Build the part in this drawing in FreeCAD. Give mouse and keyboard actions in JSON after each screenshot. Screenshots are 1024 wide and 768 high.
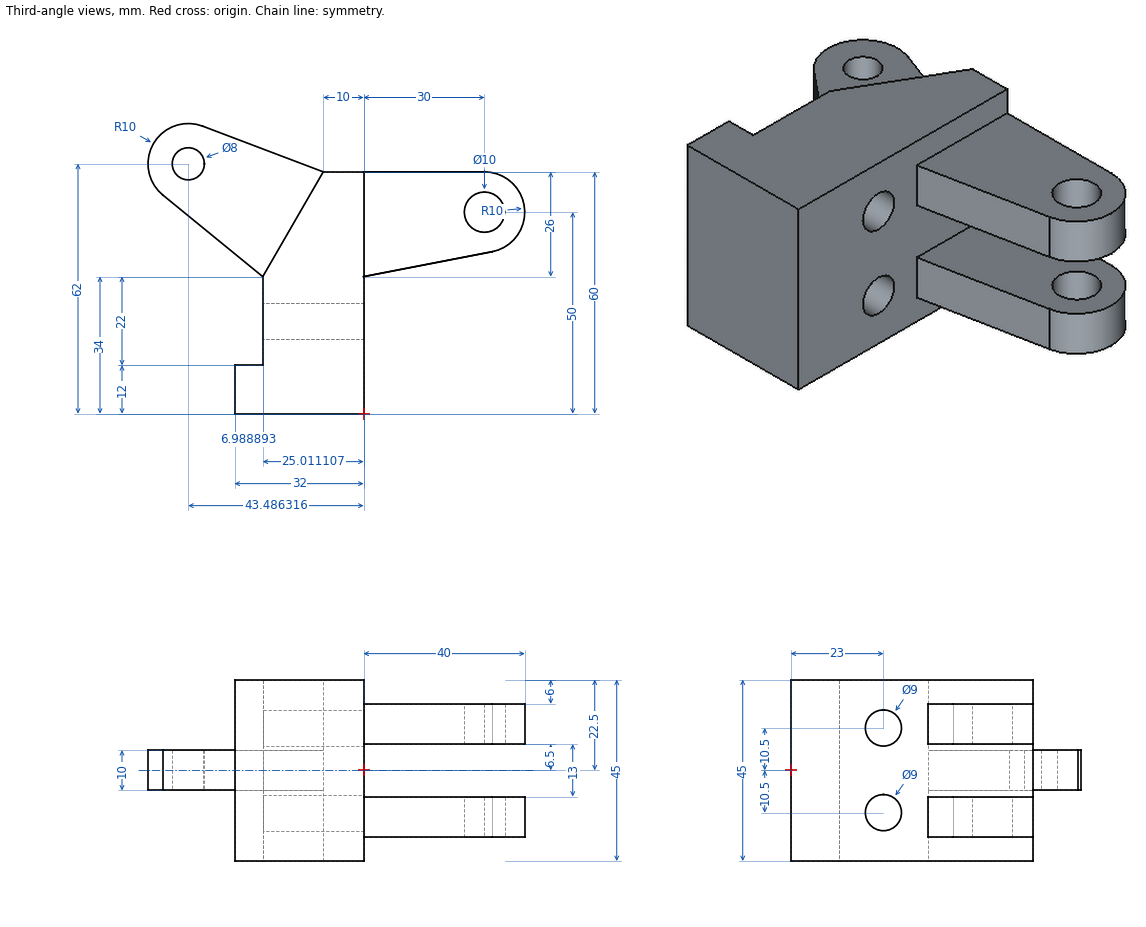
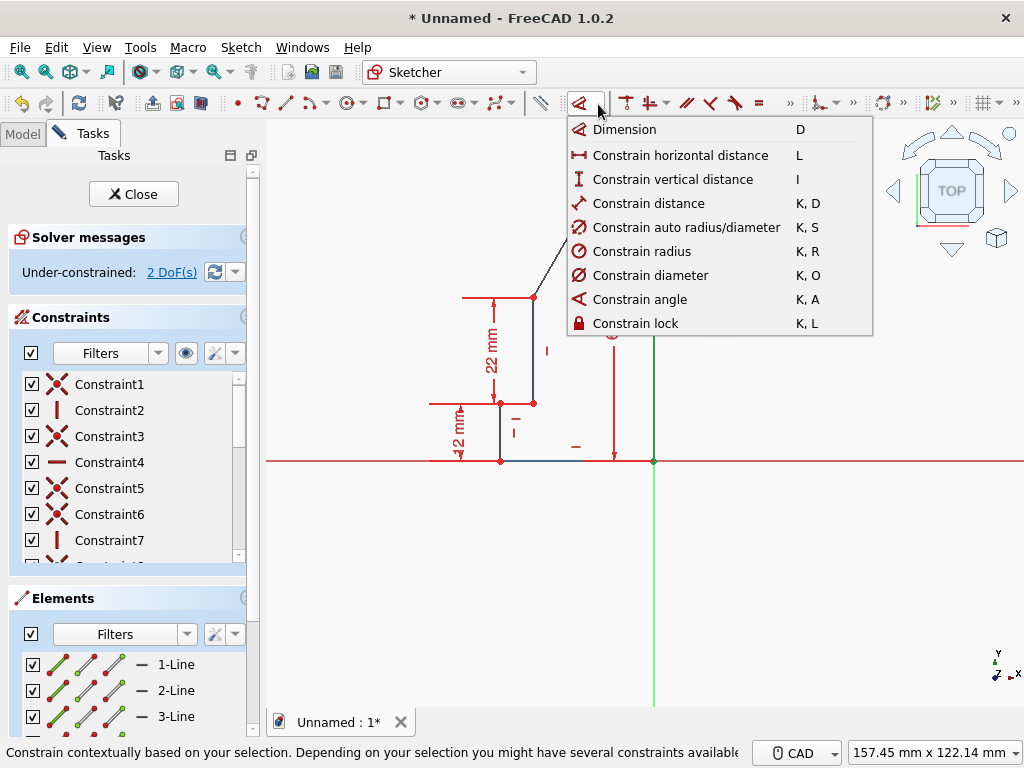
{"action": "left_click", "coordinate": [720, 155]}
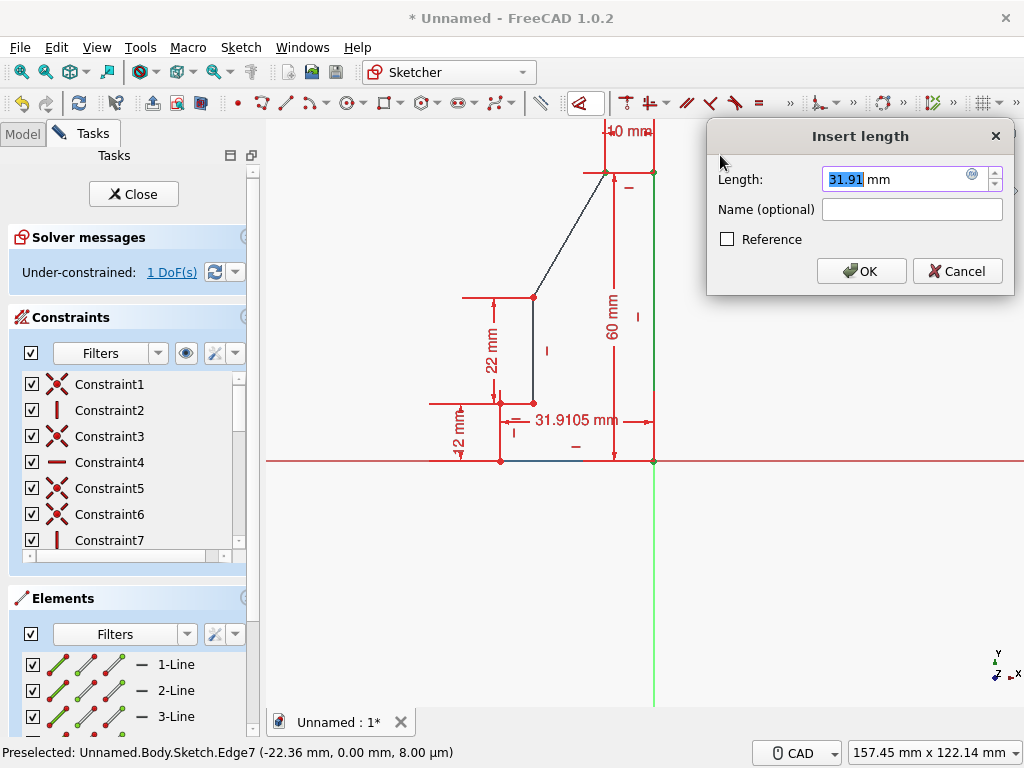
{"action": "type", "text": "32"}
{"action": "key", "text": "Return"}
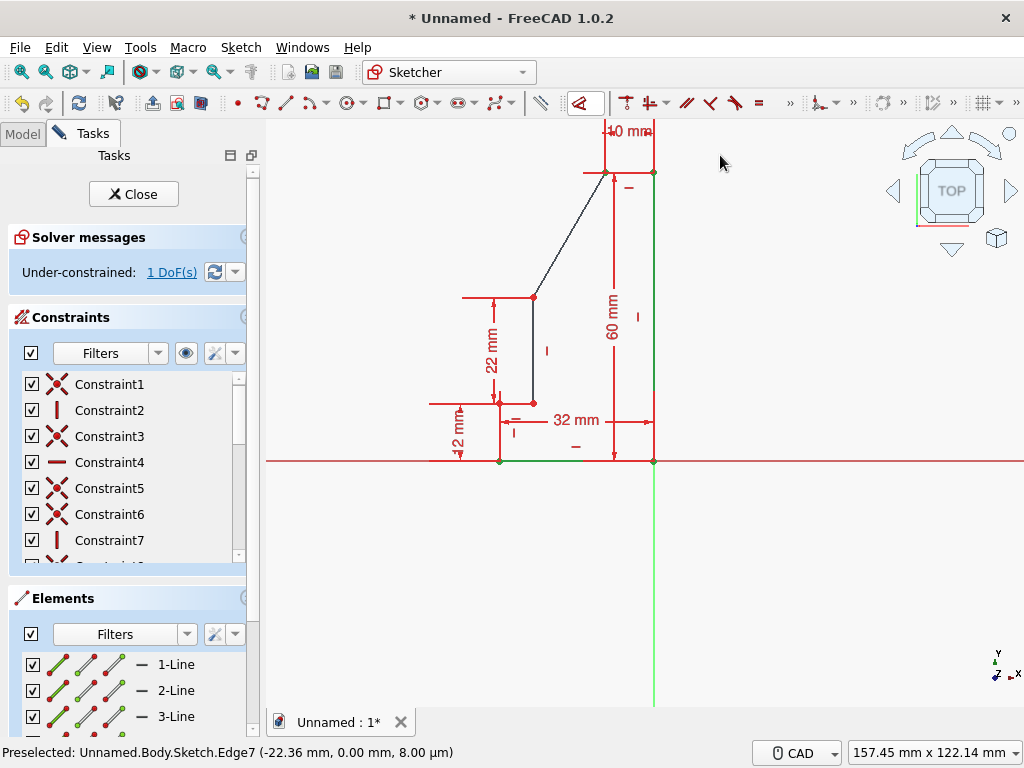
{"action": "scroll", "coordinate": [523, 404], "scroll_direction": "up", "scroll_amount": 2}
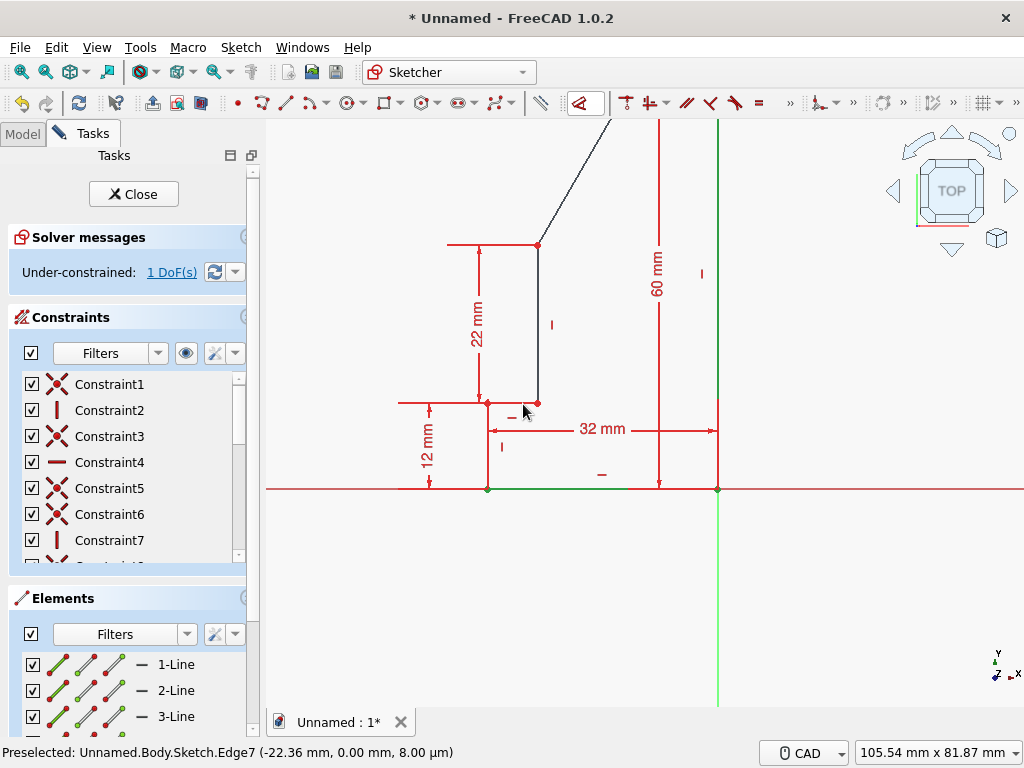
{"action": "left_click", "coordinate": [523, 403]}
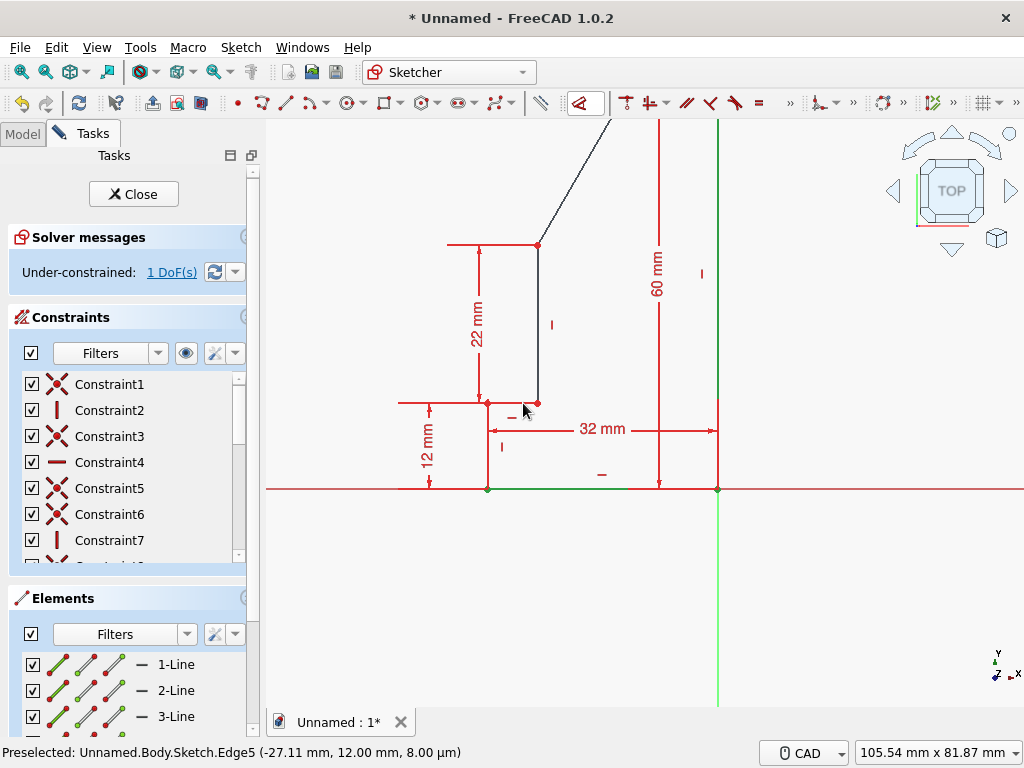
{"action": "key", "text": "l"}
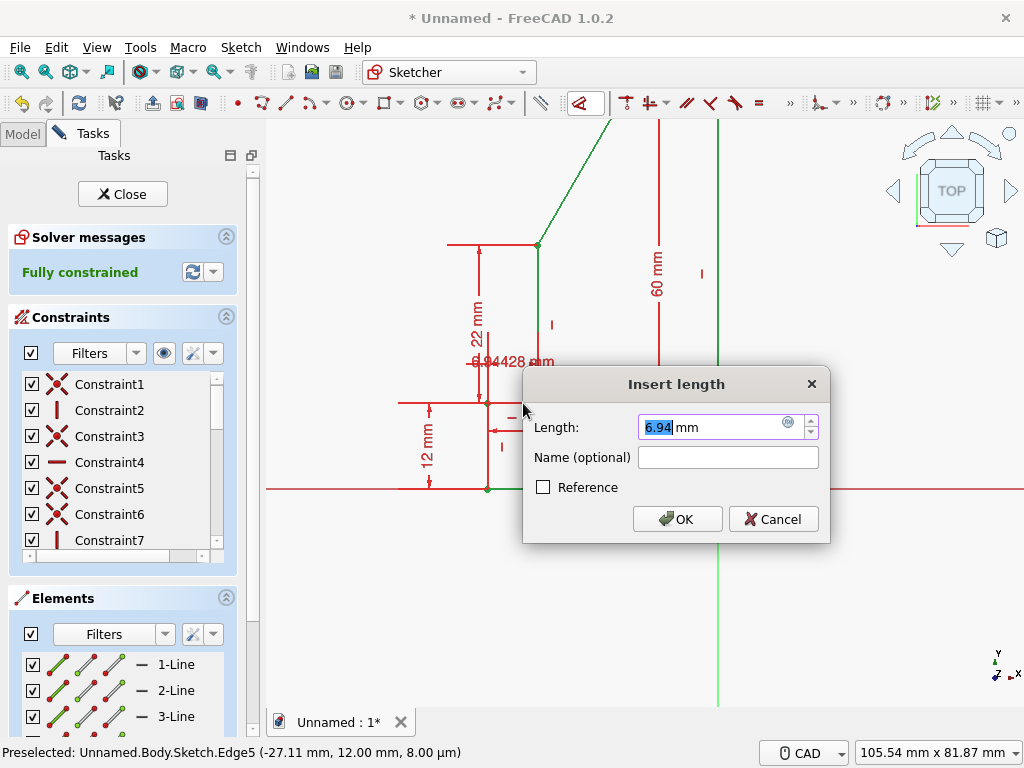
{"action": "type", "text": "6.988893"}
{"action": "key", "text": "Return"}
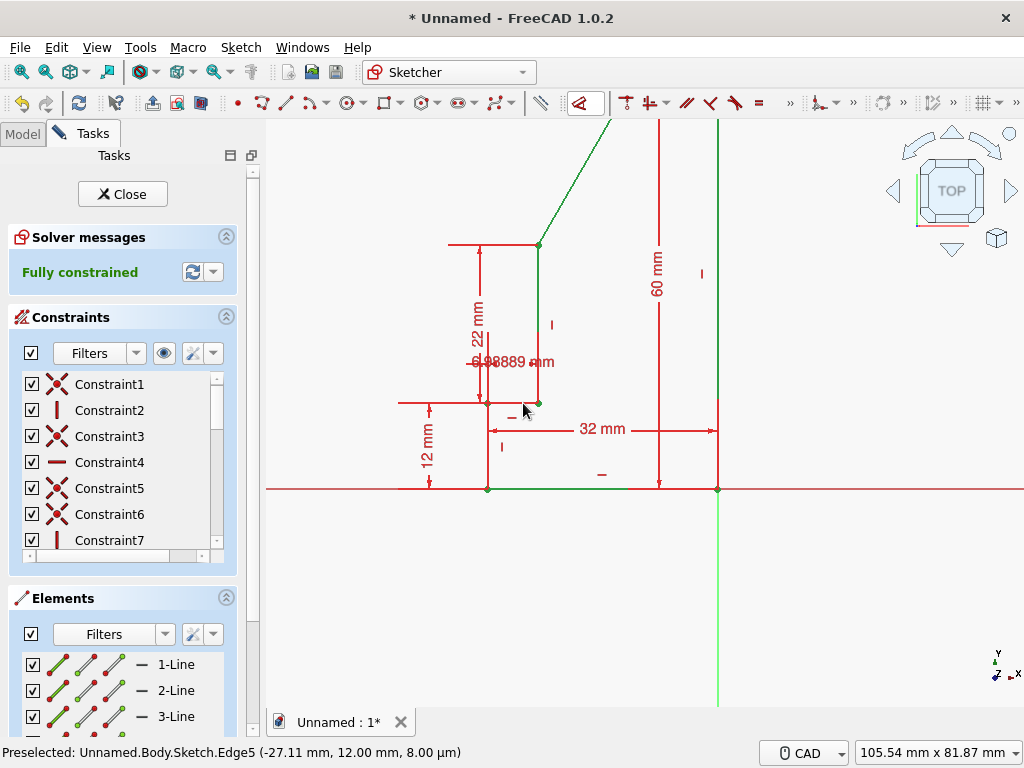
{"action": "left_click", "coordinate": [123, 194]}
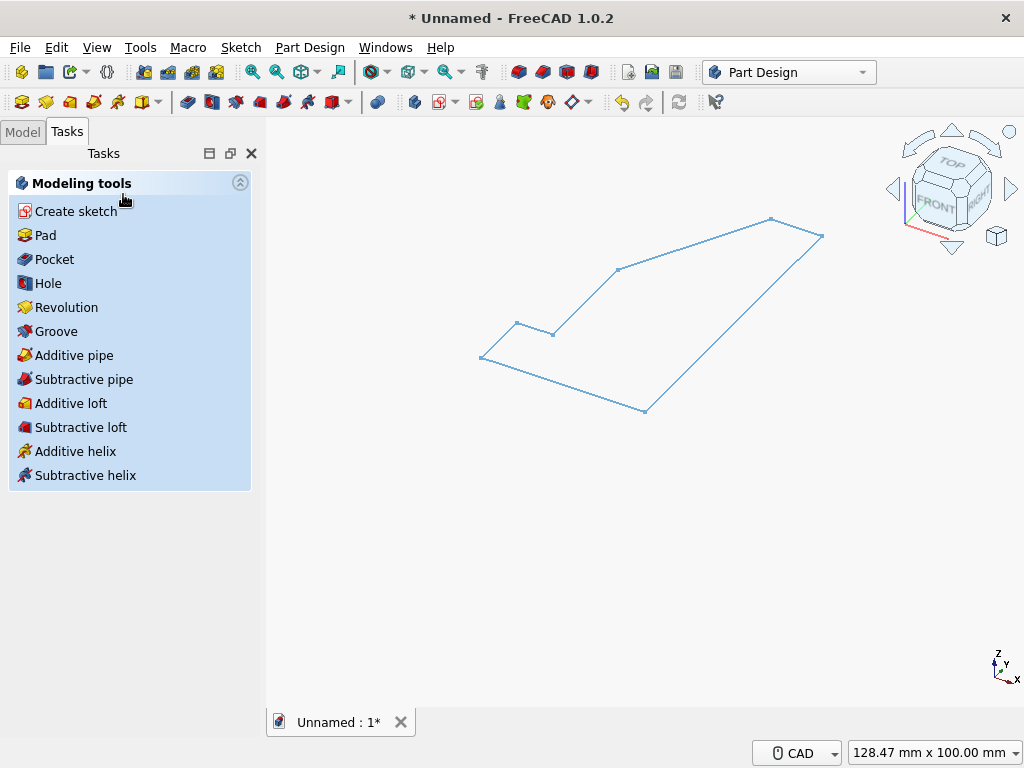
{"action": "left_click", "coordinate": [22, 102]}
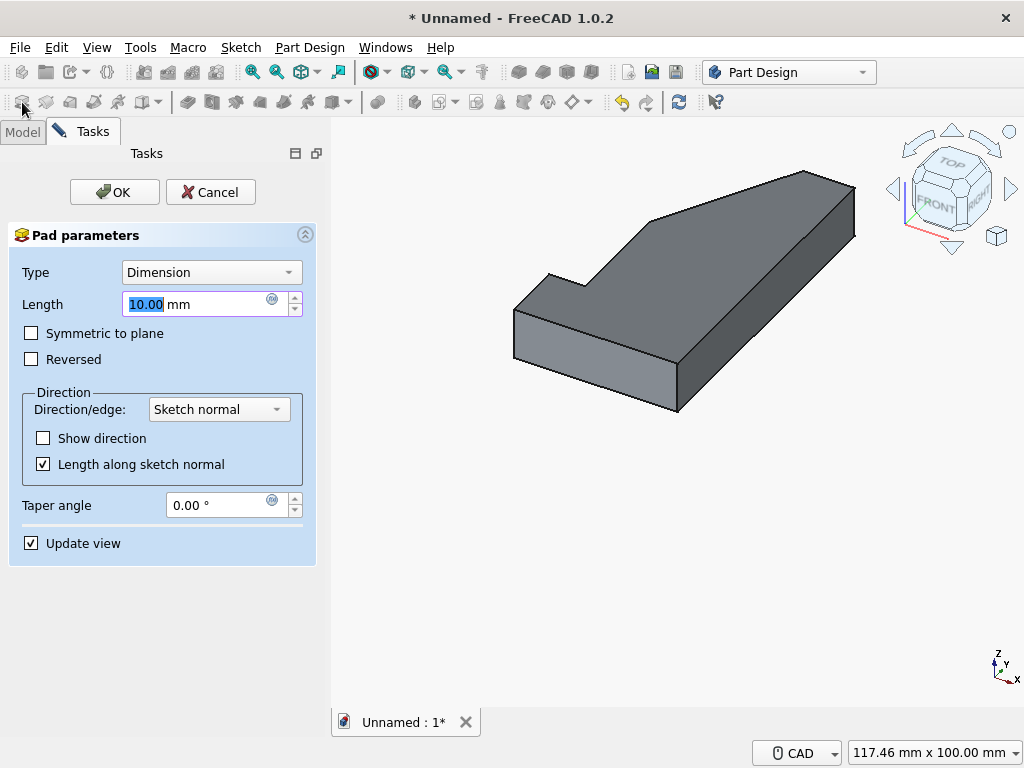
{"action": "type", "text": "45"}
{"action": "key", "text": "Tab"}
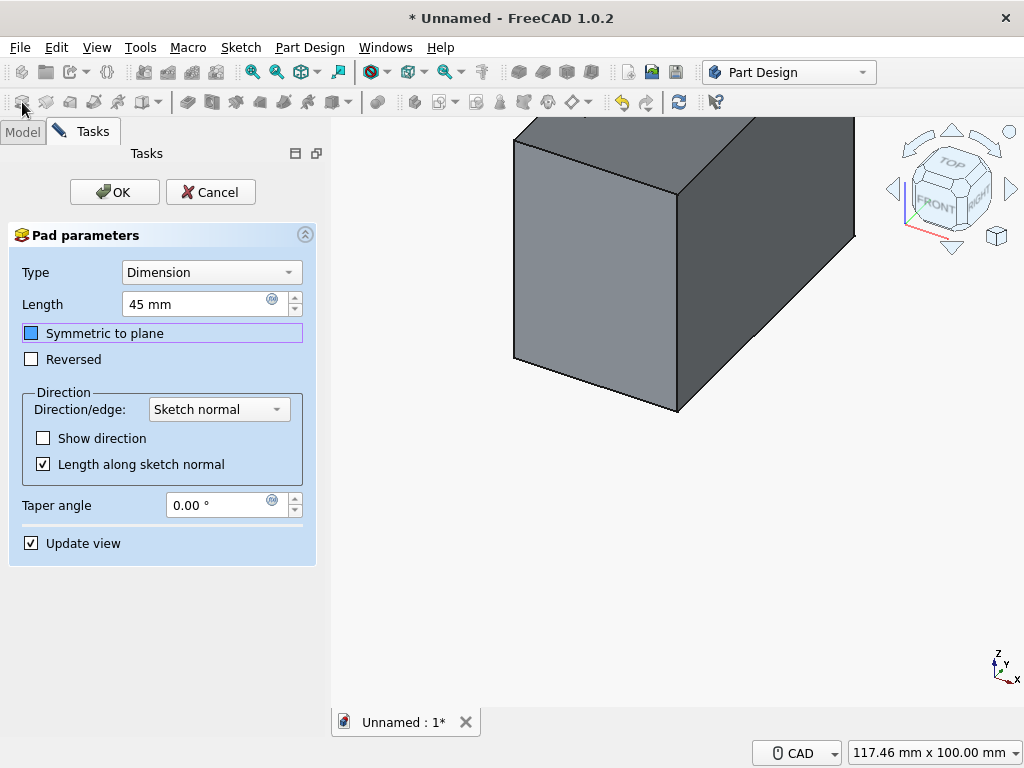
{"action": "left_click", "coordinate": [30, 333]}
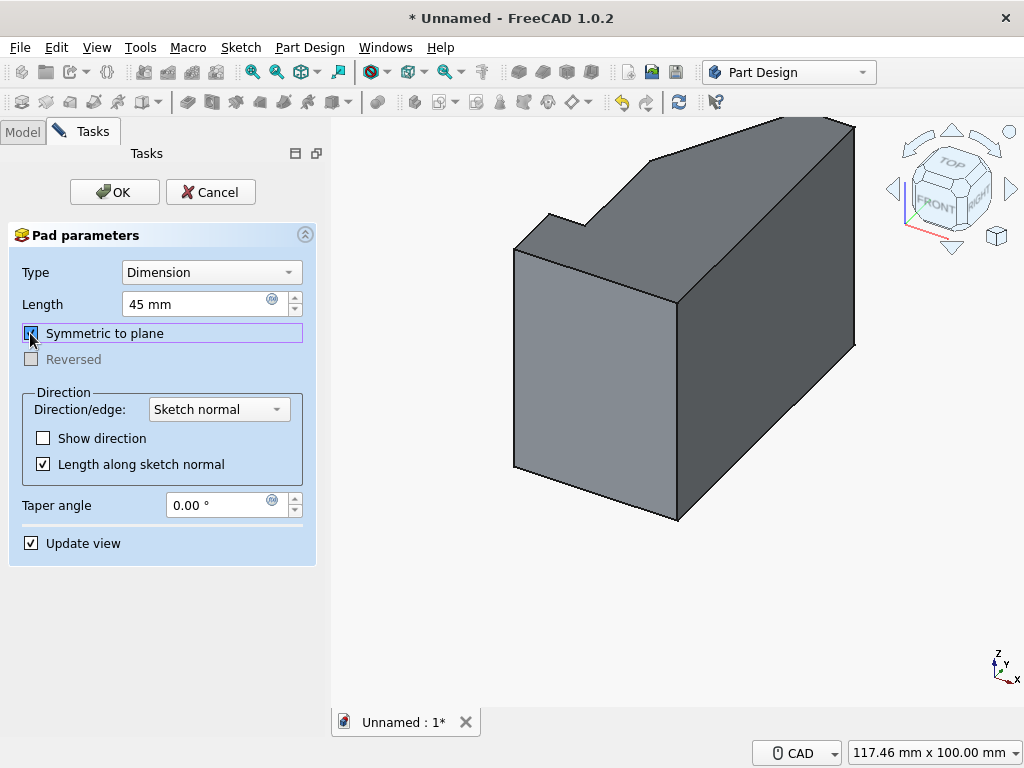
{"action": "left_click", "coordinate": [115, 192]}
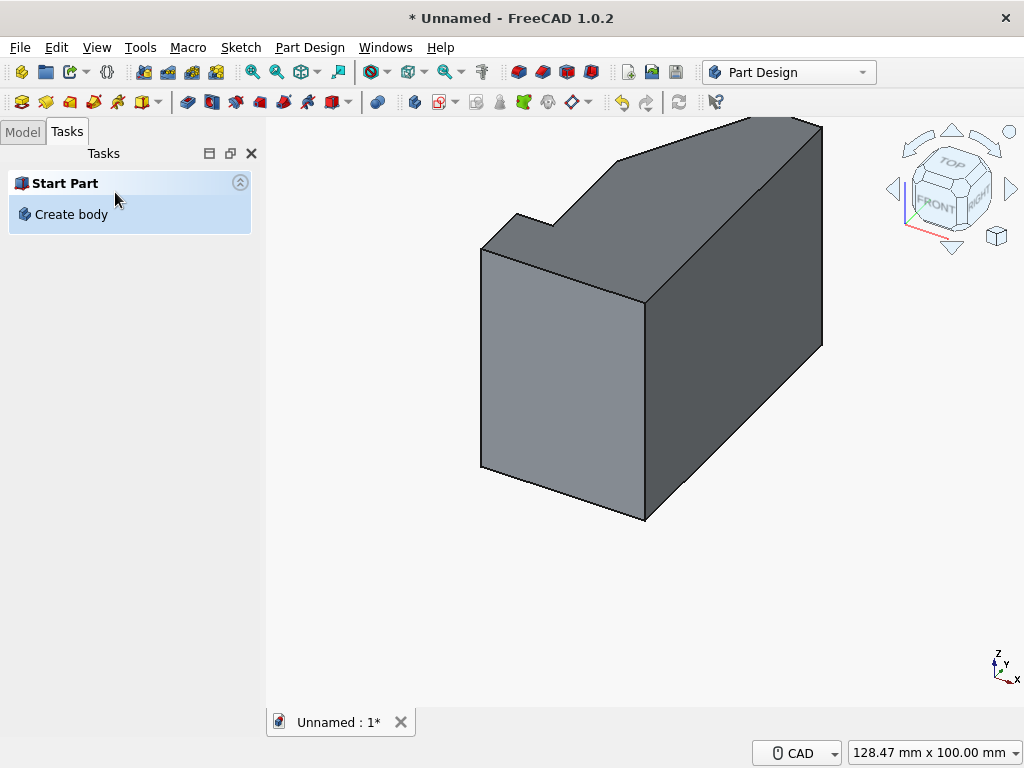
{"action": "key", "text": "v f"}